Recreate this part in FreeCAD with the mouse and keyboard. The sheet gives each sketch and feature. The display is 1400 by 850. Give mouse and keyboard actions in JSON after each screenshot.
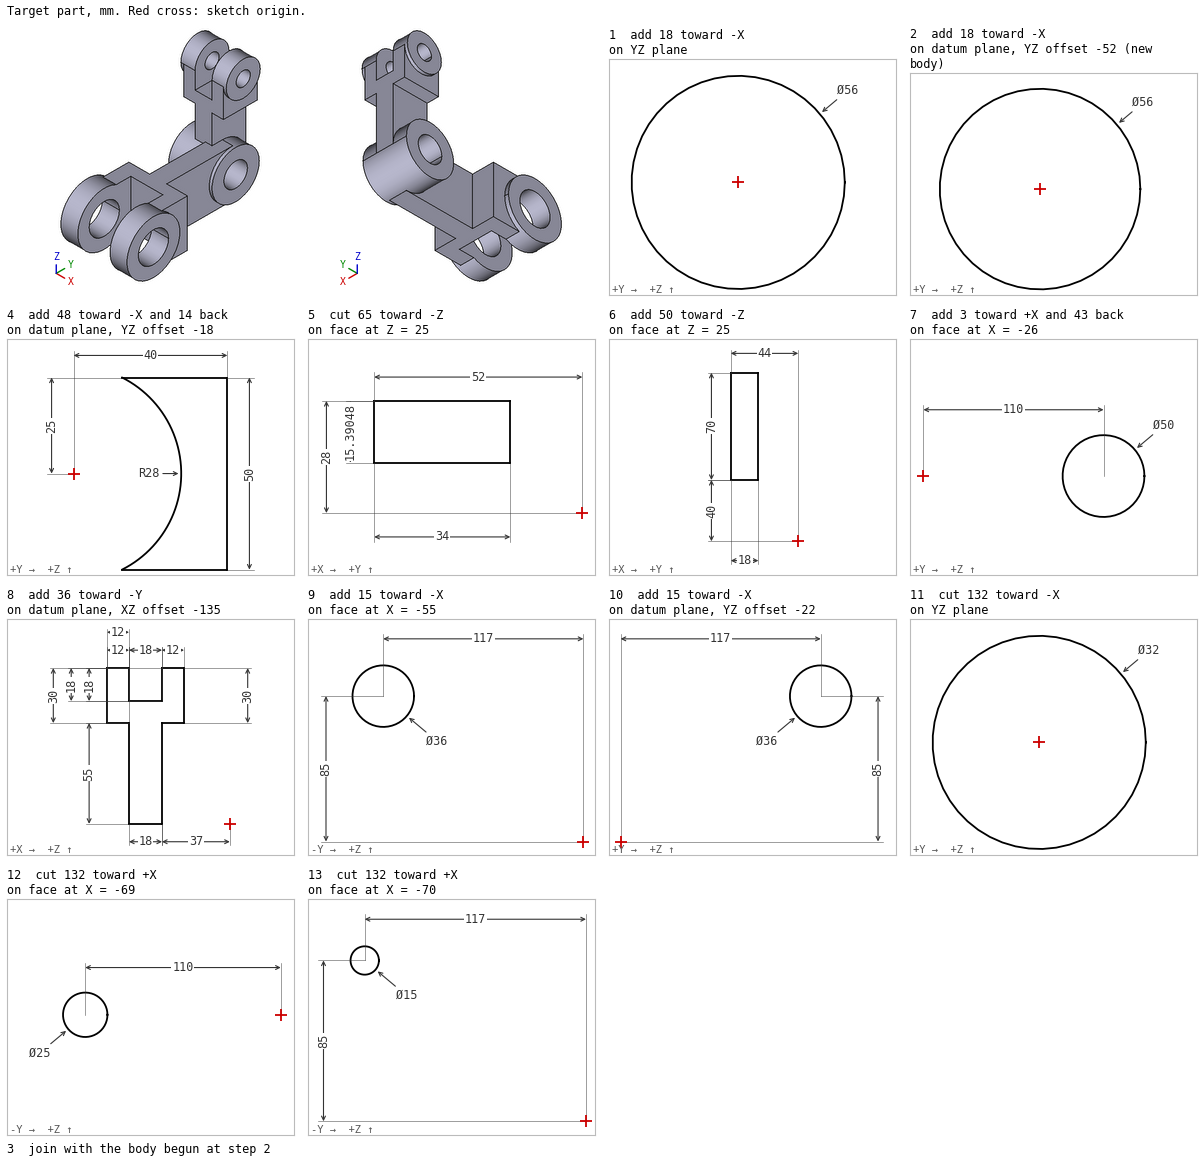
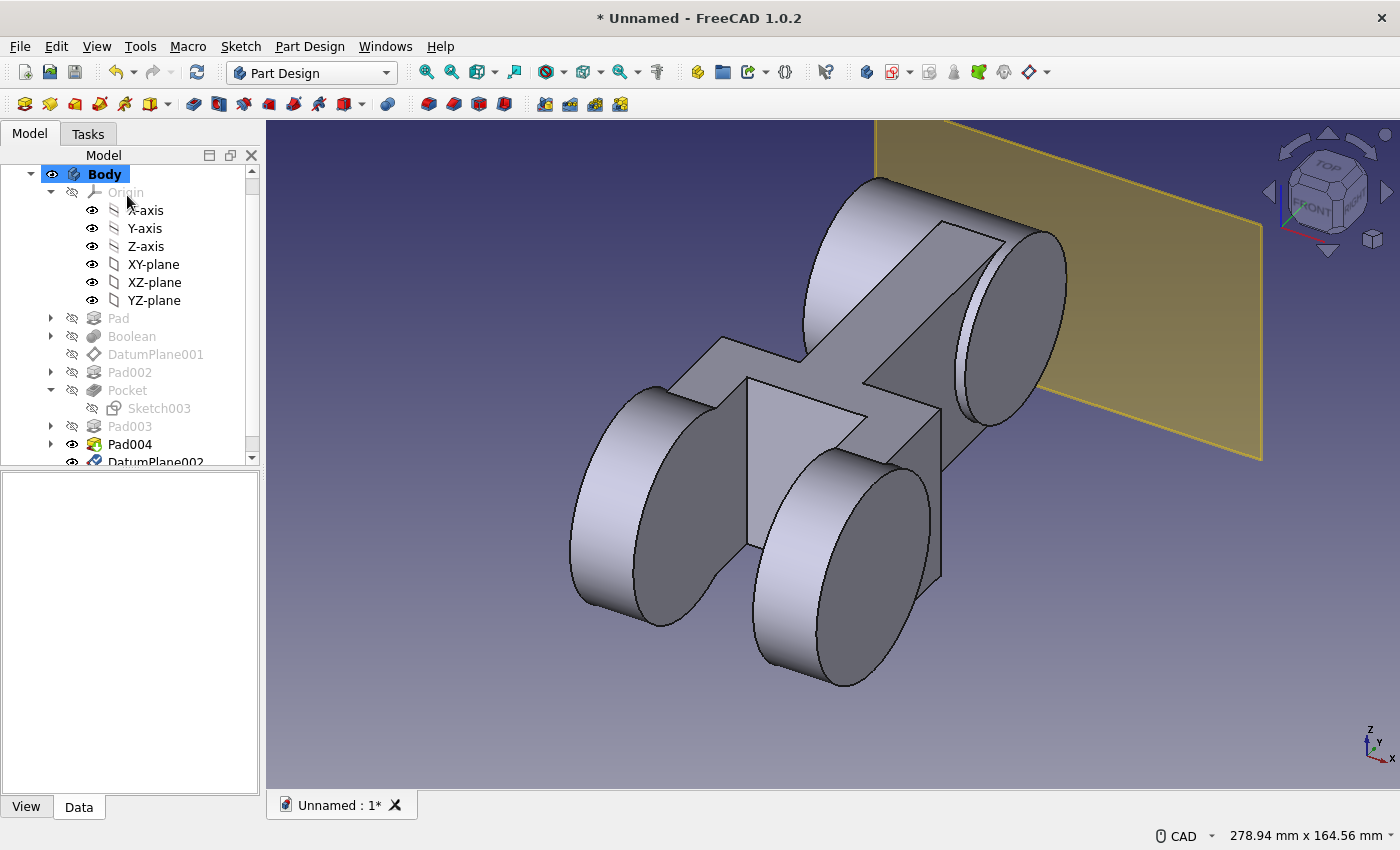
{"action": "left_click", "coordinate": [117, 462]}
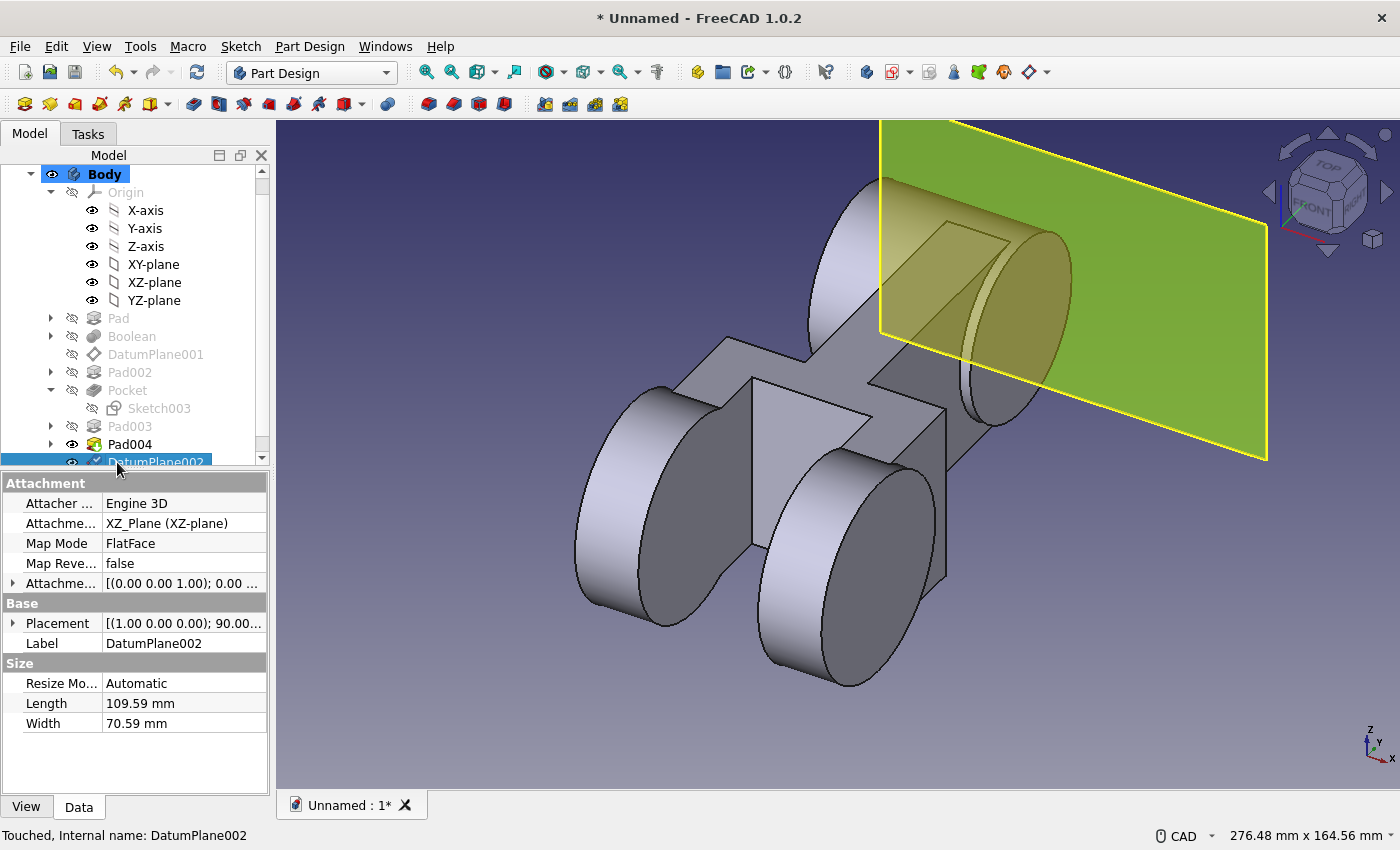
{"action": "left_click", "coordinate": [892, 72]}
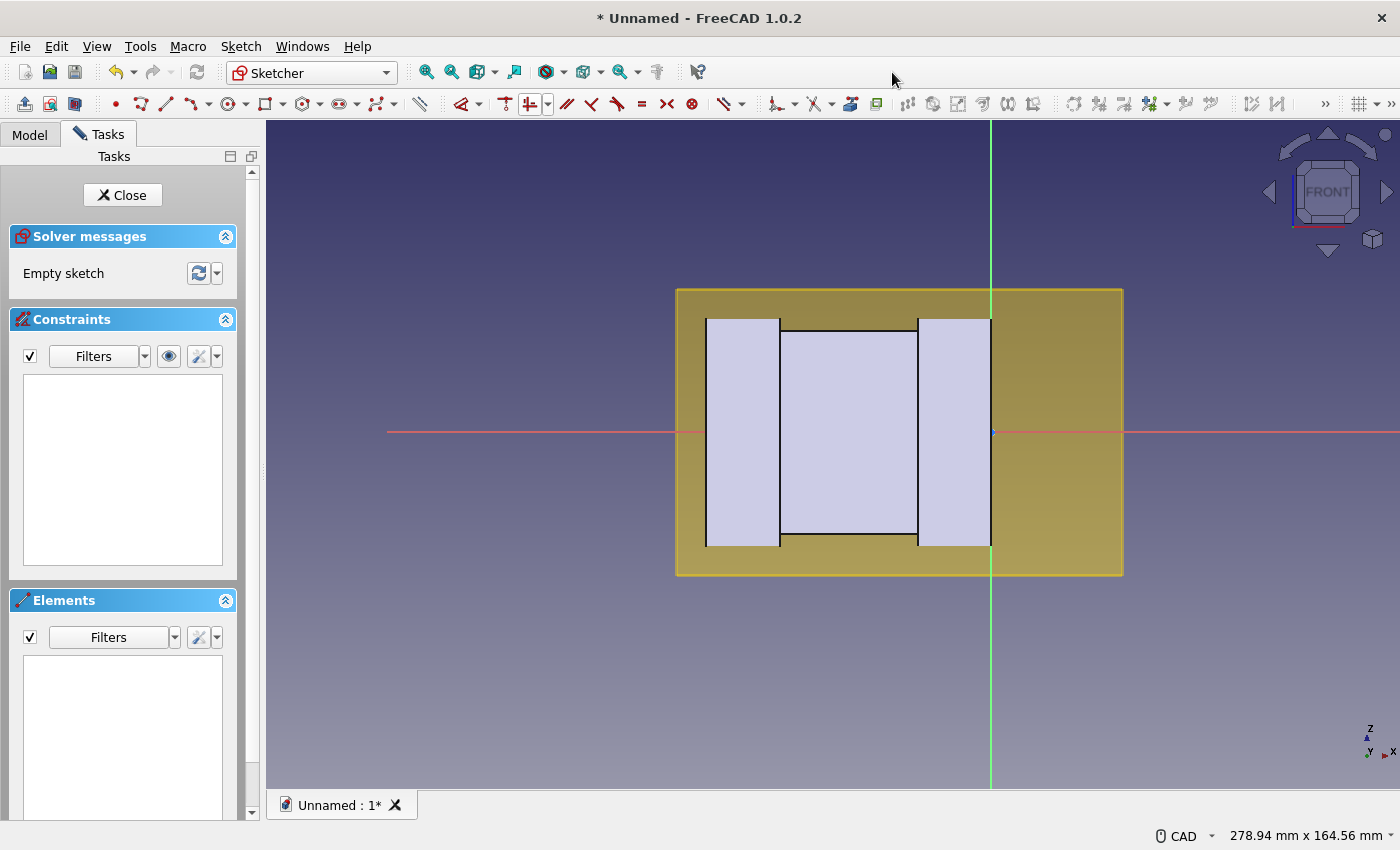
{"action": "key", "text": "q s"}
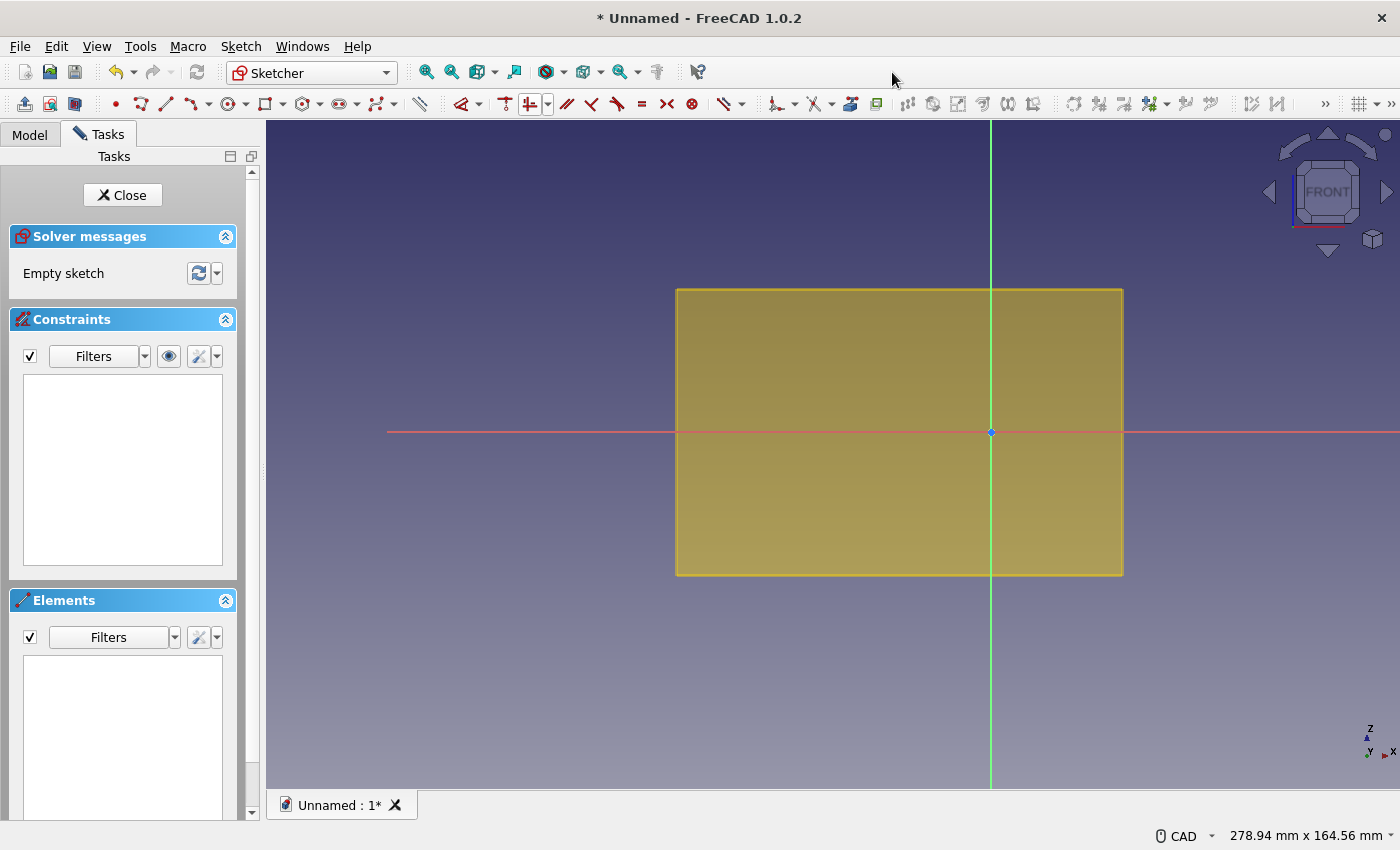
{"action": "scroll", "coordinate": [357, 761], "scroll_direction": "down", "scroll_amount": 1}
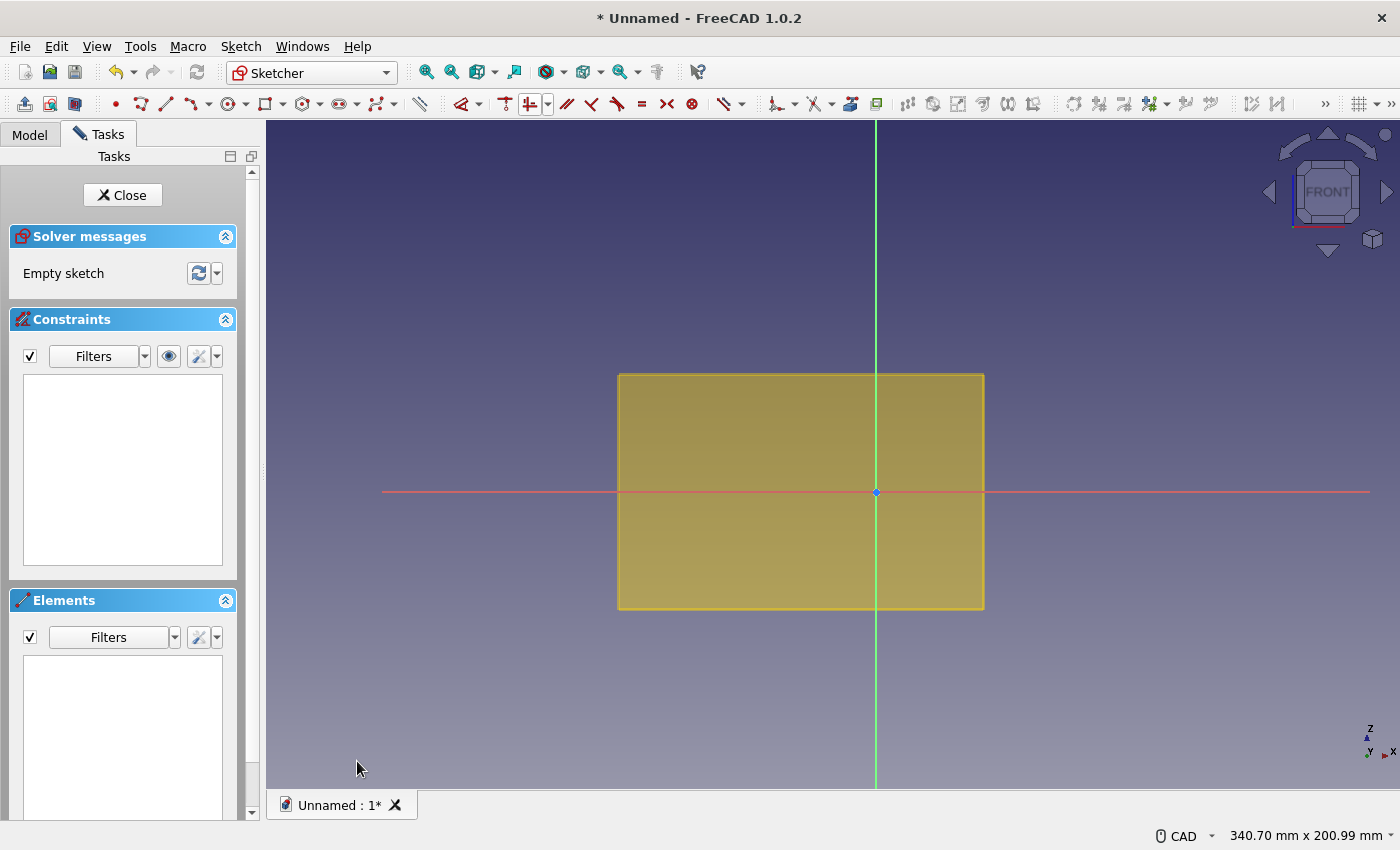
{"action": "scroll", "coordinate": [765, 148], "scroll_direction": "up", "scroll_amount": 2}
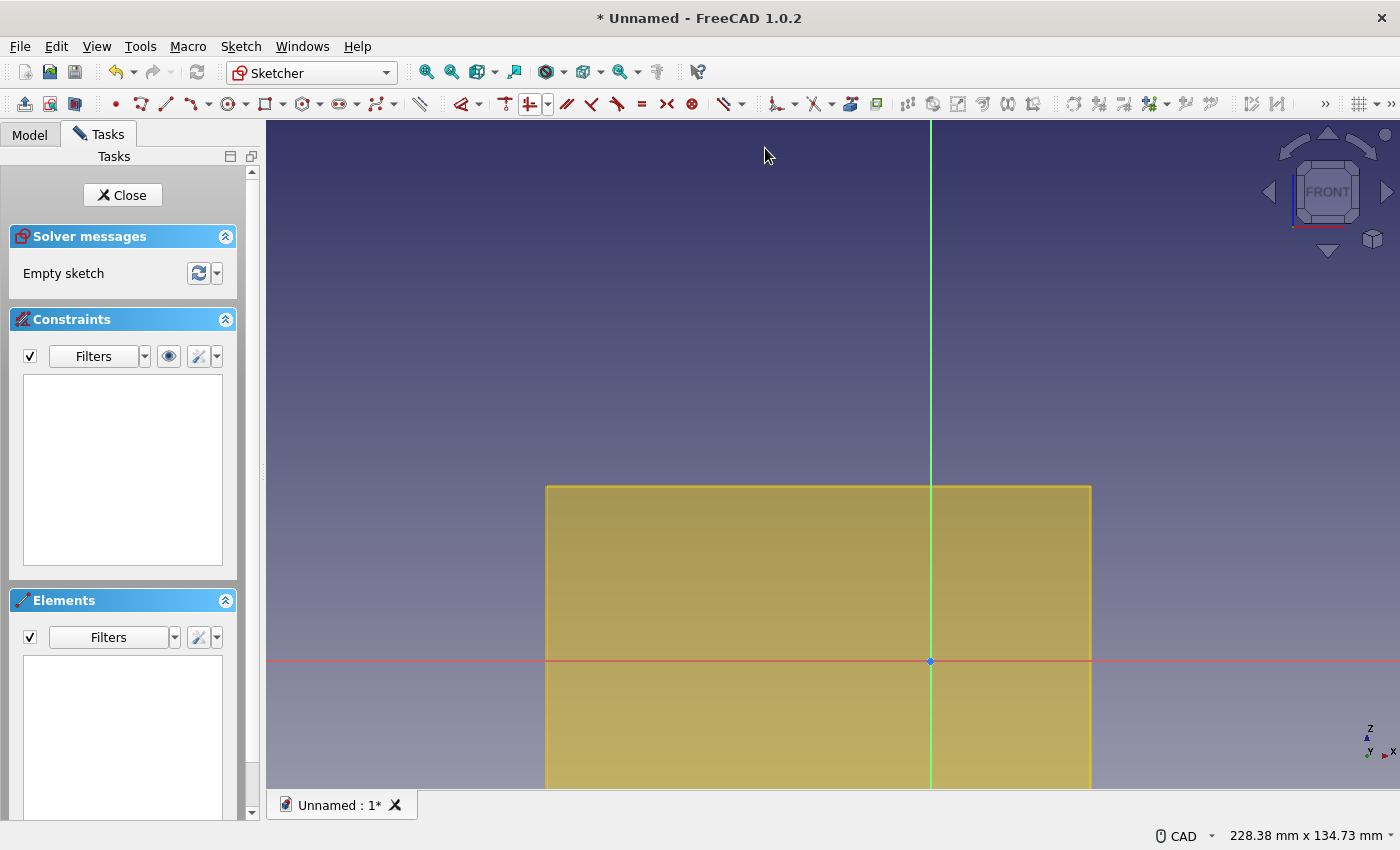
{"action": "left_click", "coordinate": [141, 104]}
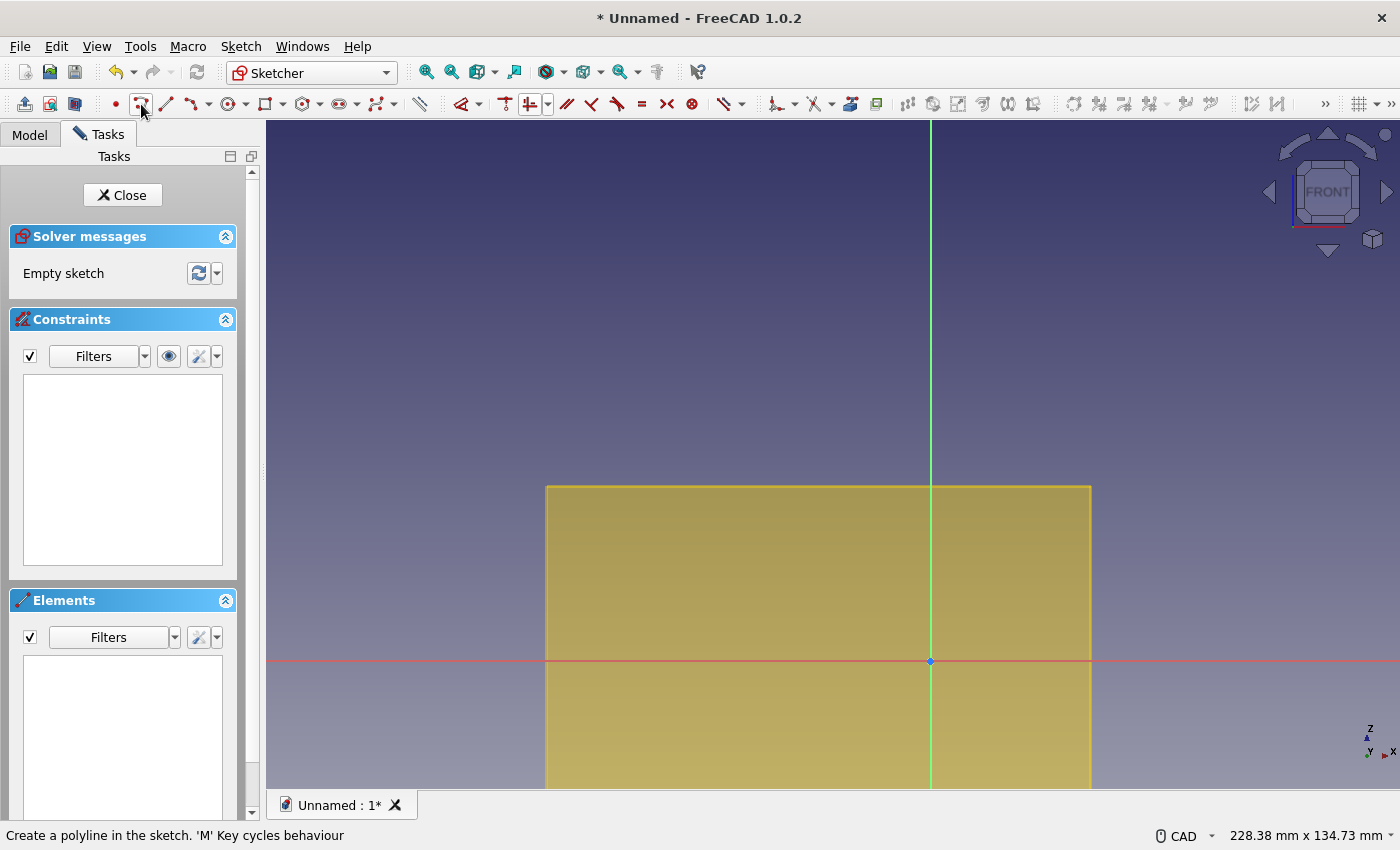
{"action": "left_click", "coordinate": [747, 661]}
{"action": "left_click", "coordinate": [657, 652]}
{"action": "left_click", "coordinate": [657, 388]}
{"action": "left_click", "coordinate": [598, 388]}
{"action": "left_click", "coordinate": [598, 239]}
{"action": "left_click", "coordinate": [657, 239]}
{"action": "left_click", "coordinate": [657, 329]}
{"action": "left_click", "coordinate": [747, 329]}
{"action": "left_click", "coordinate": [747, 239]}
{"action": "left_click", "coordinate": [806, 239]}
{"action": "left_click", "coordinate": [806, 388]}
{"action": "left_click", "coordinate": [747, 388]}
{"action": "left_click", "coordinate": [747, 661]}
{"action": "key", "text": "Escape"}
{"action": "key", "text": "Escape"}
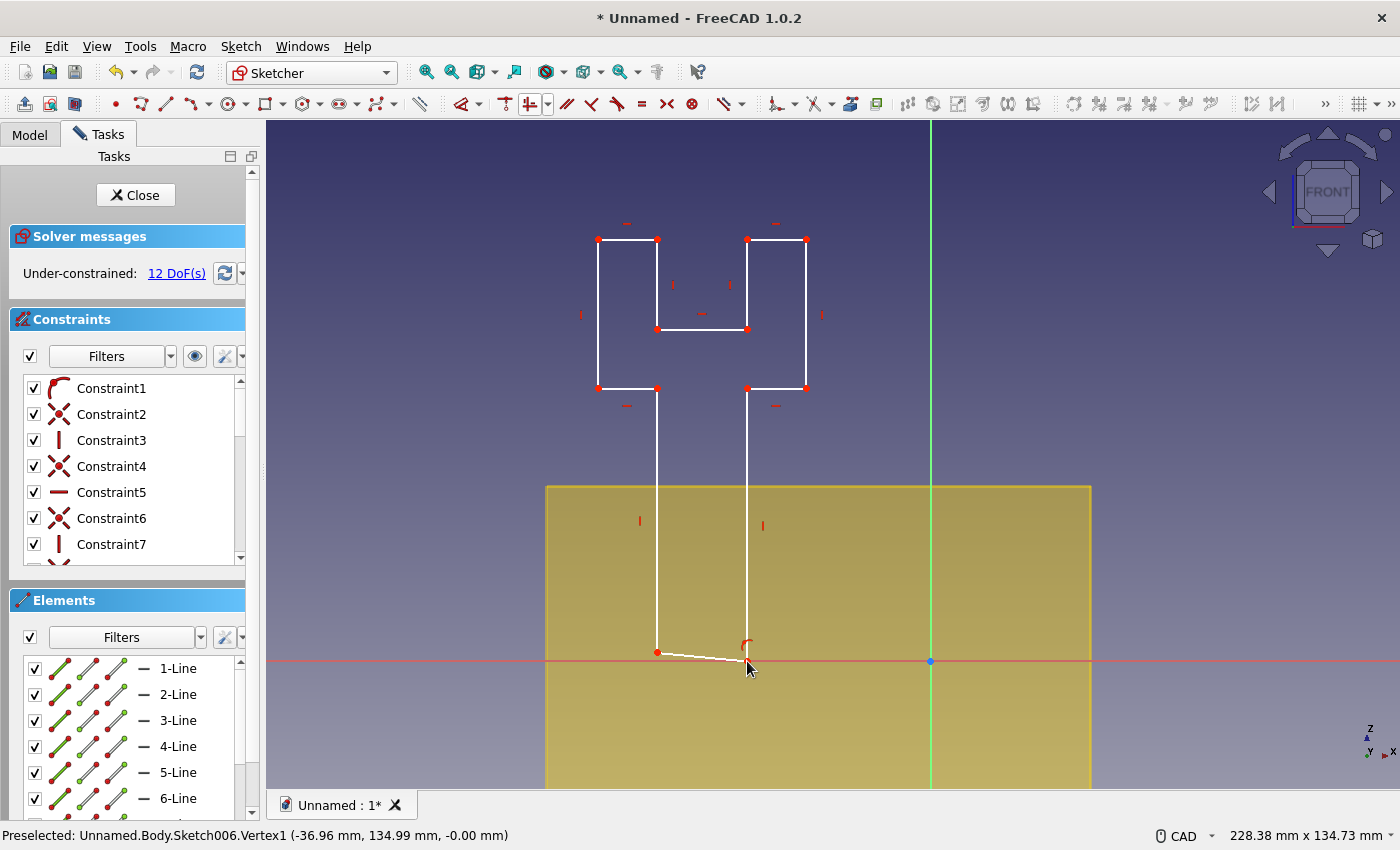
{"action": "left_click", "coordinate": [720, 659]}